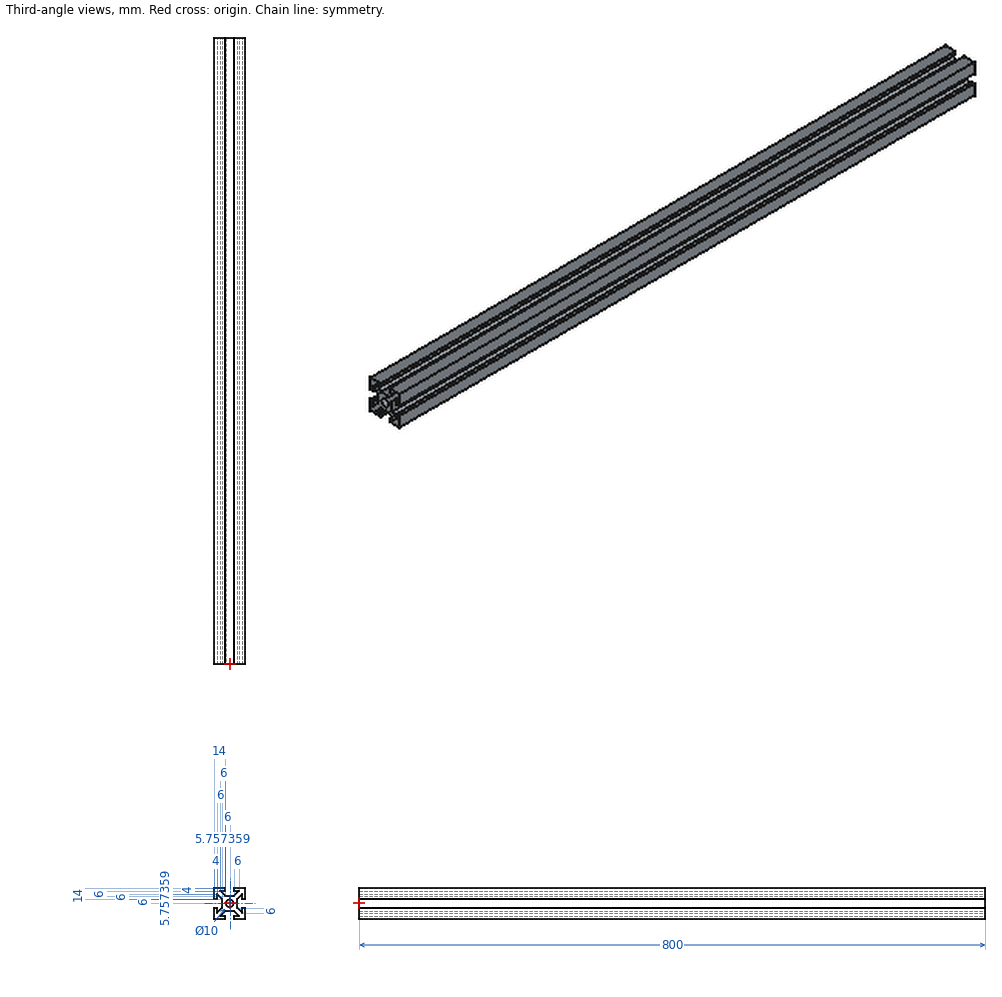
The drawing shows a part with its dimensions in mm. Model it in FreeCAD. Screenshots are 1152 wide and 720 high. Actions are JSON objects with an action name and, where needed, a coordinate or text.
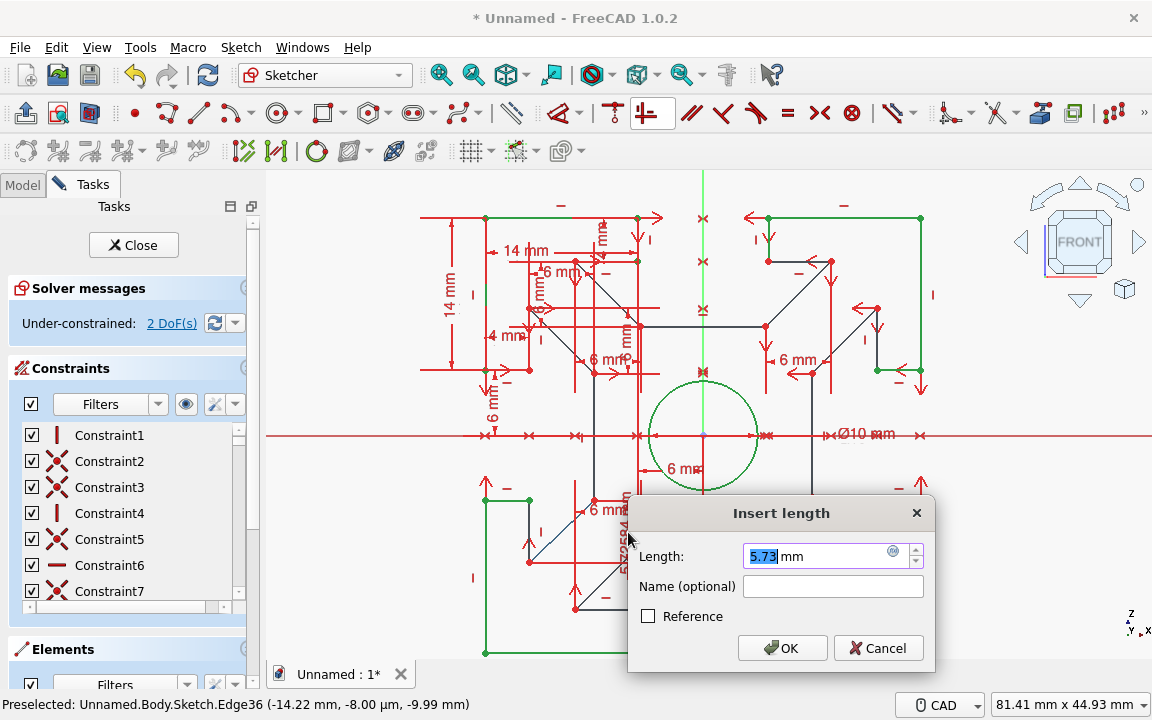
{"action": "type", "text": "6"}
{"action": "key", "text": "Return"}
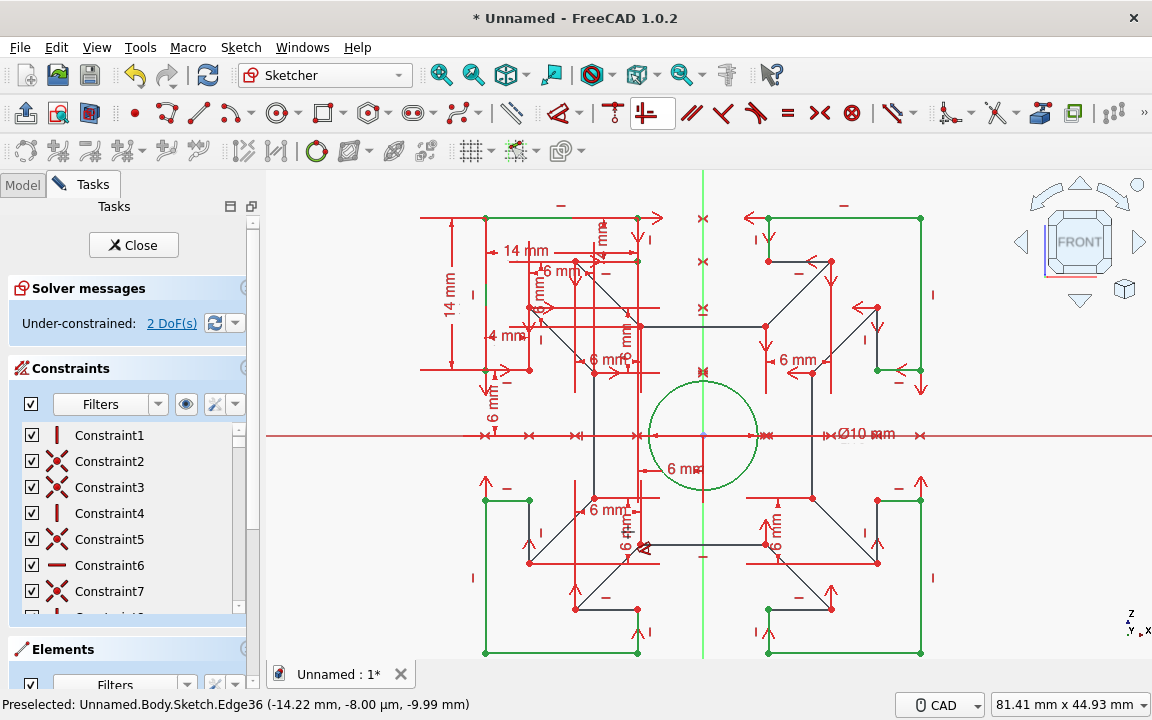
{"action": "left_click", "coordinate": [529, 327]}
{"action": "left_click", "coordinate": [471, 361]}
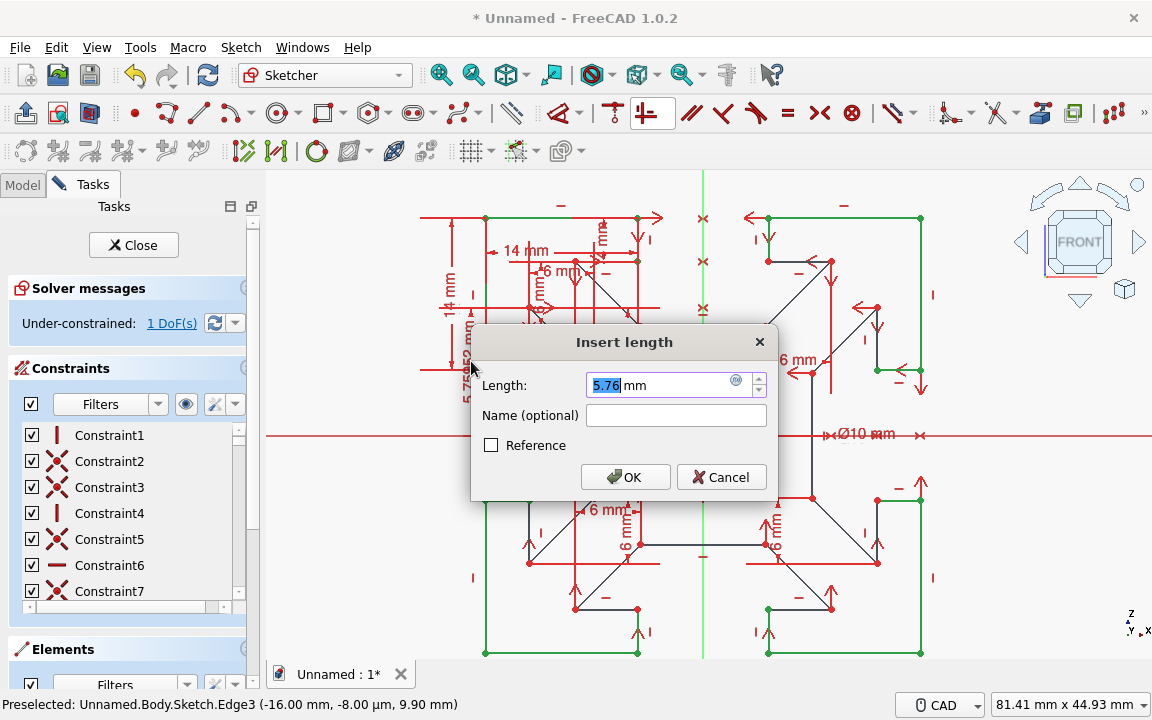
{"action": "type", "text": "5.757359"}
{"action": "key", "text": "Return"}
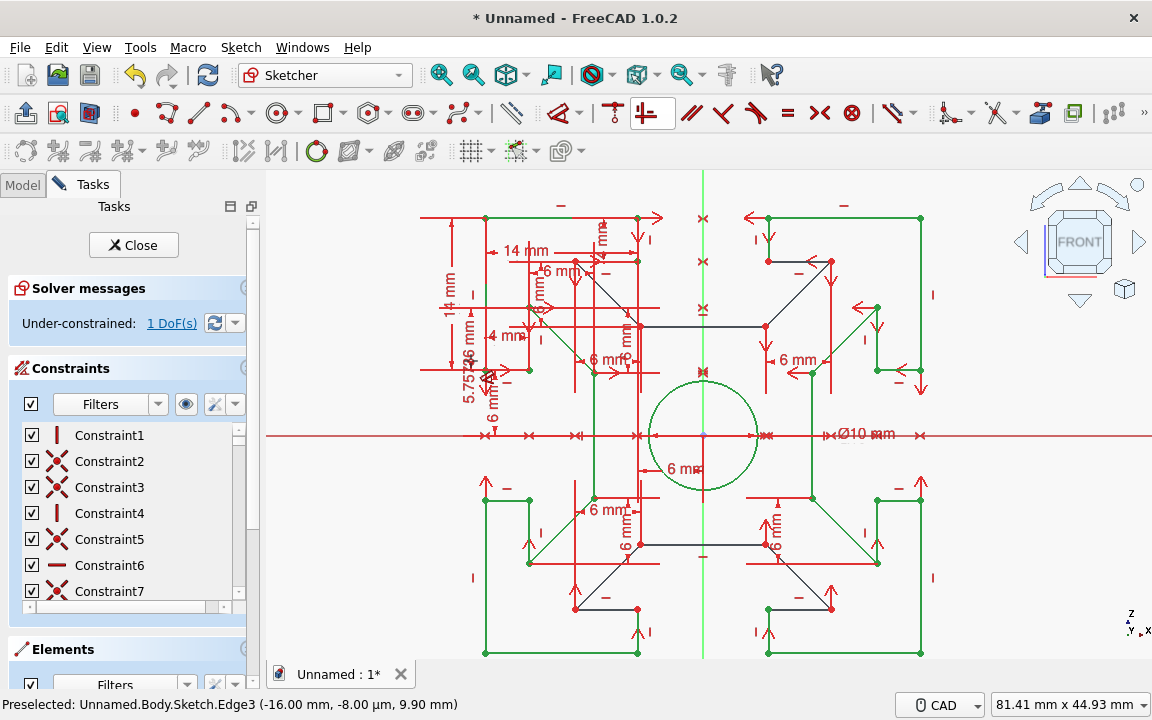
{"action": "left_click", "coordinate": [619, 262]}
{"action": "left_click", "coordinate": [629, 296]}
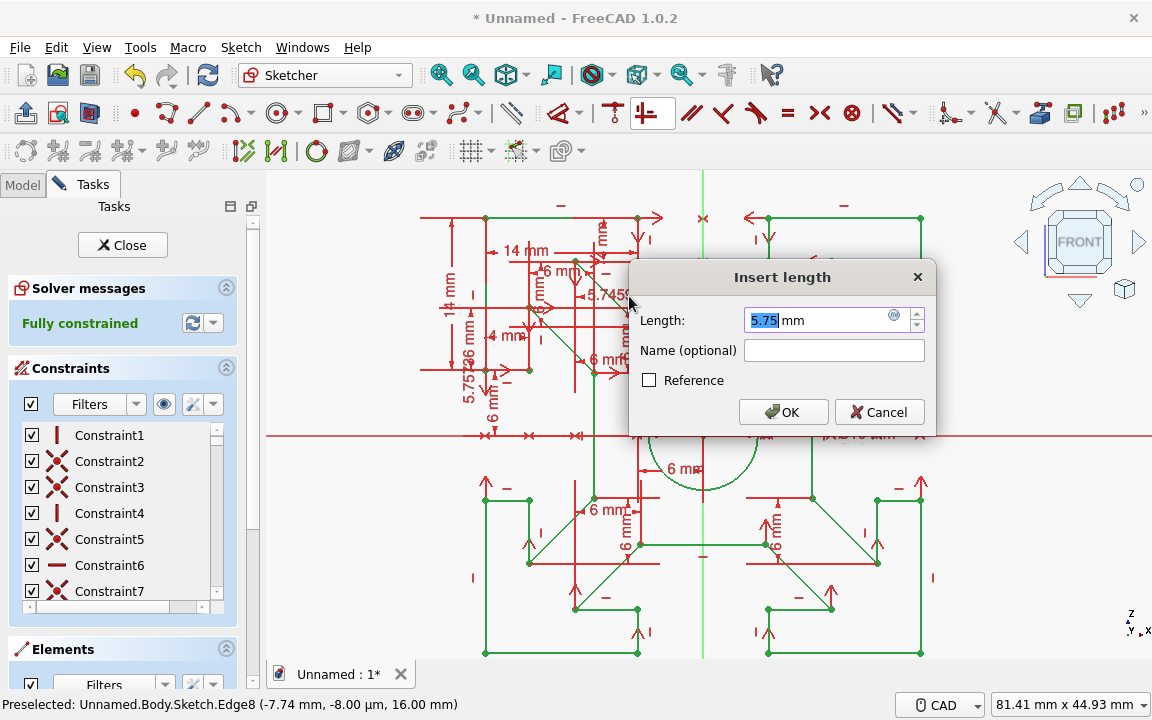
{"action": "type", "text": "5.757359"}
{"action": "key", "text": "Return"}
{"action": "key", "text": "Escape"}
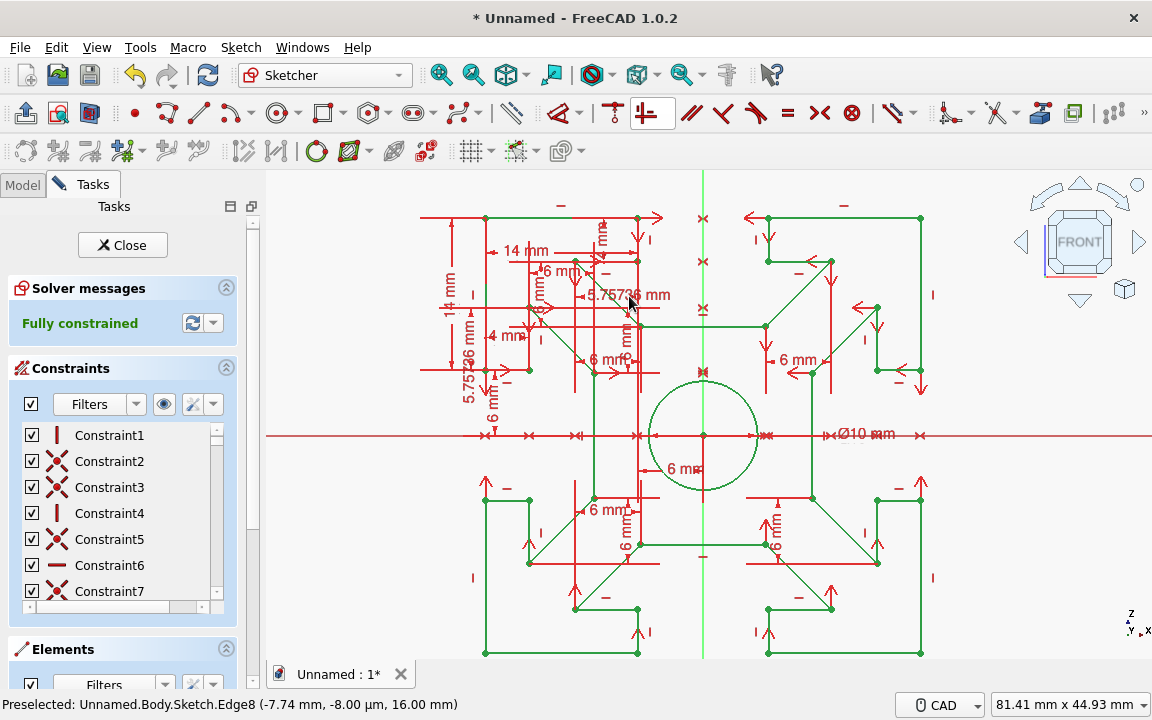
{"action": "left_click", "coordinate": [123, 245]}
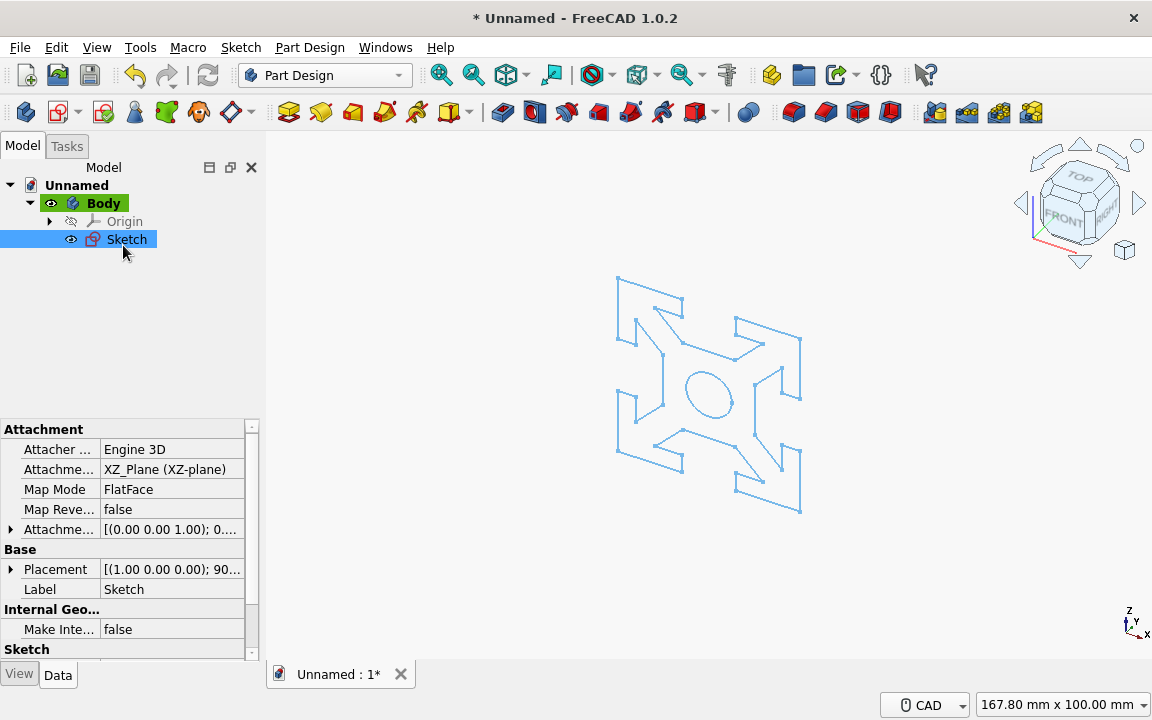
{"action": "left_click", "coordinate": [290, 112]}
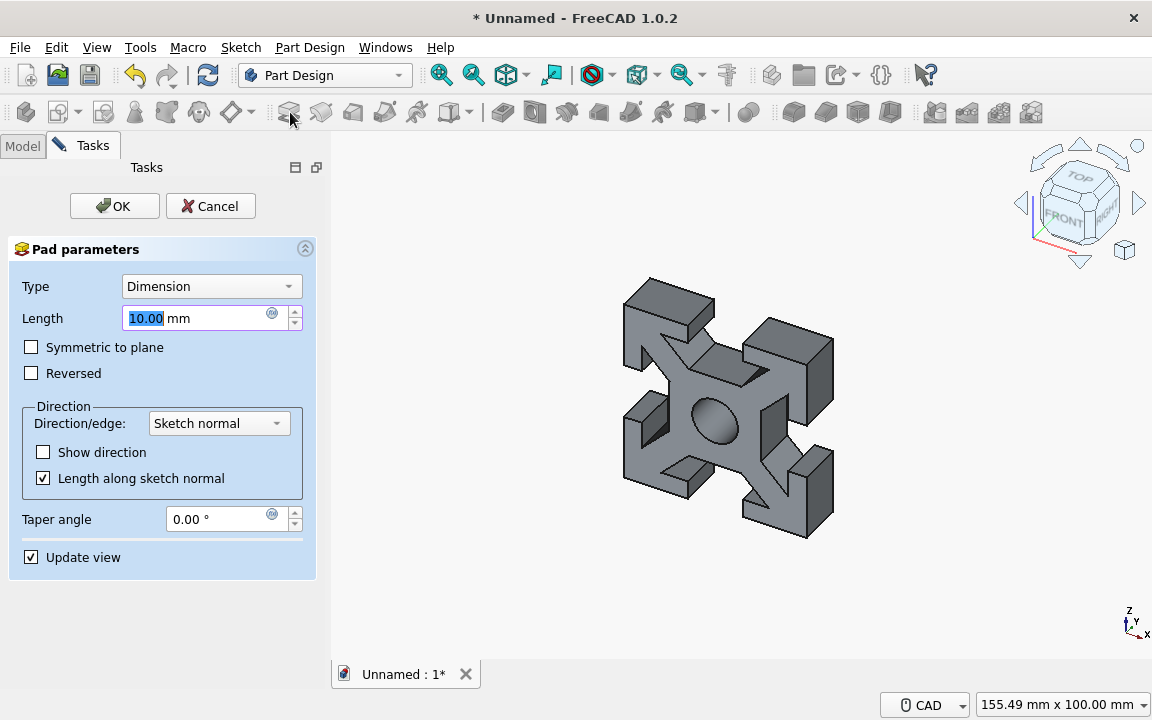
{"action": "type", "text": "800"}
{"action": "key", "text": "Tab"}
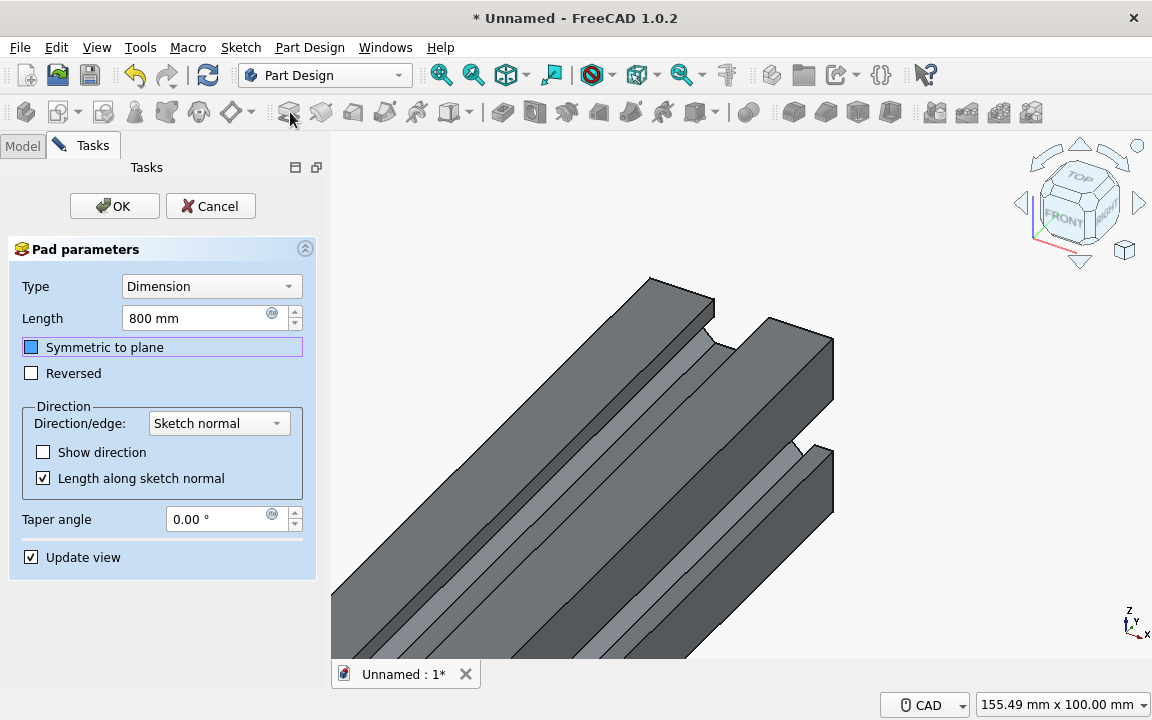
{"action": "left_click", "coordinate": [30, 373]}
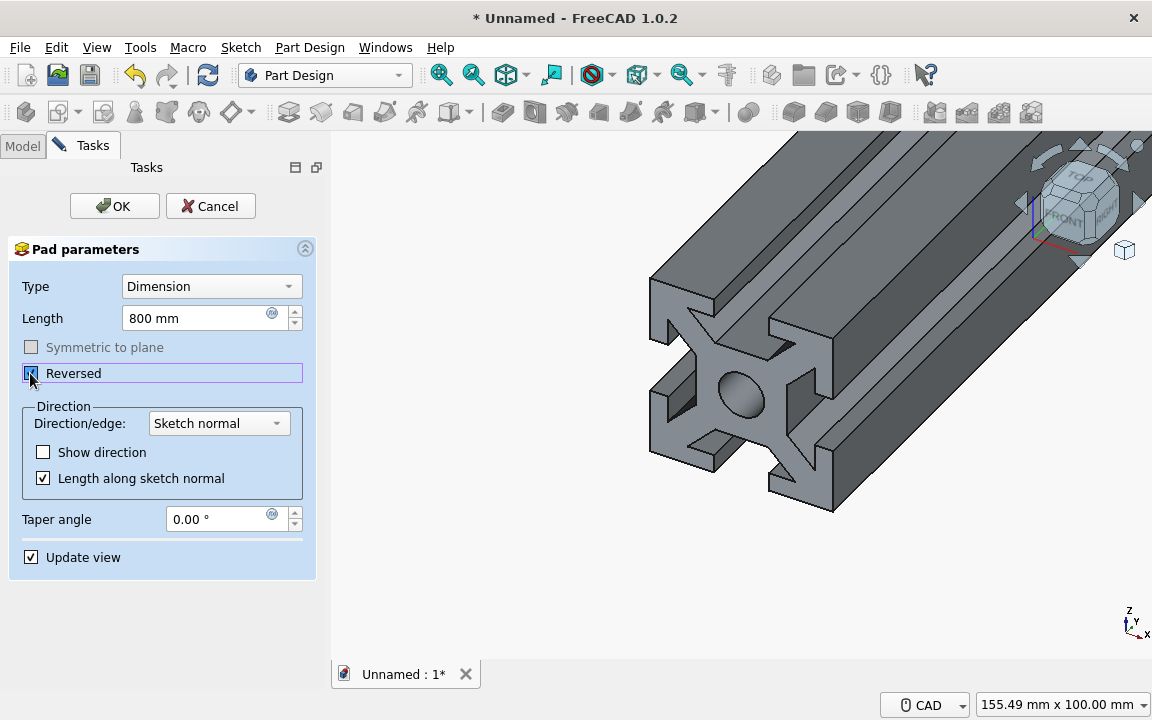
{"action": "left_click", "coordinate": [115, 206]}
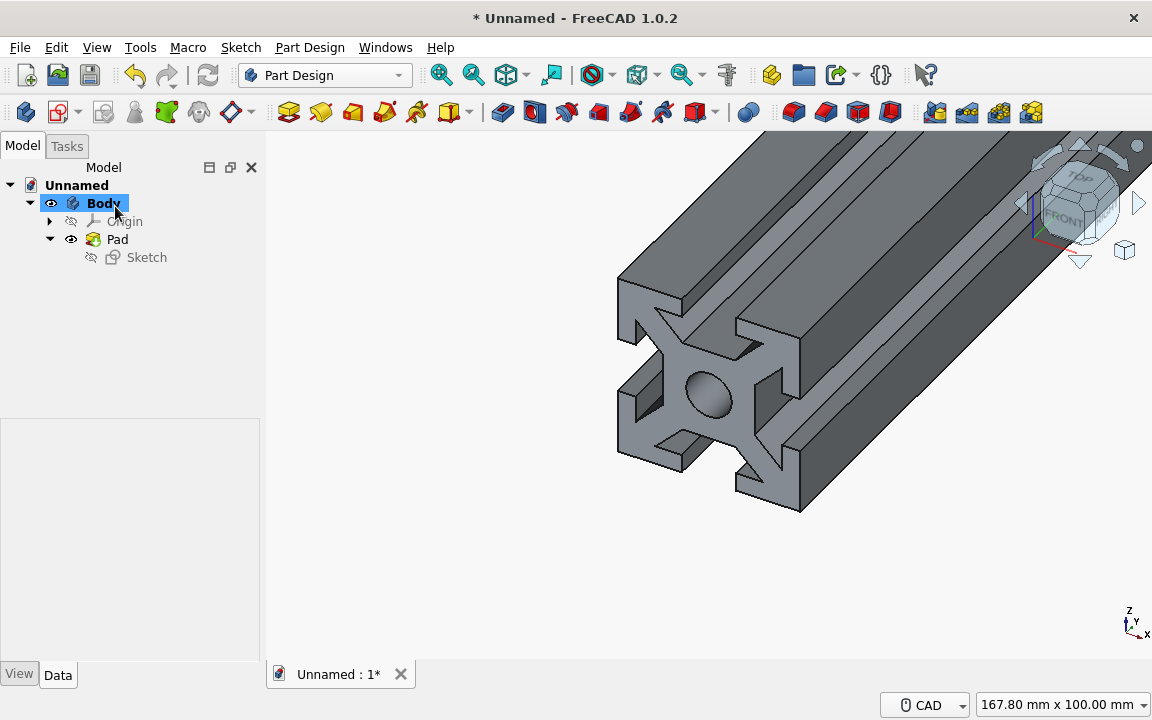
{"action": "key", "text": "0"}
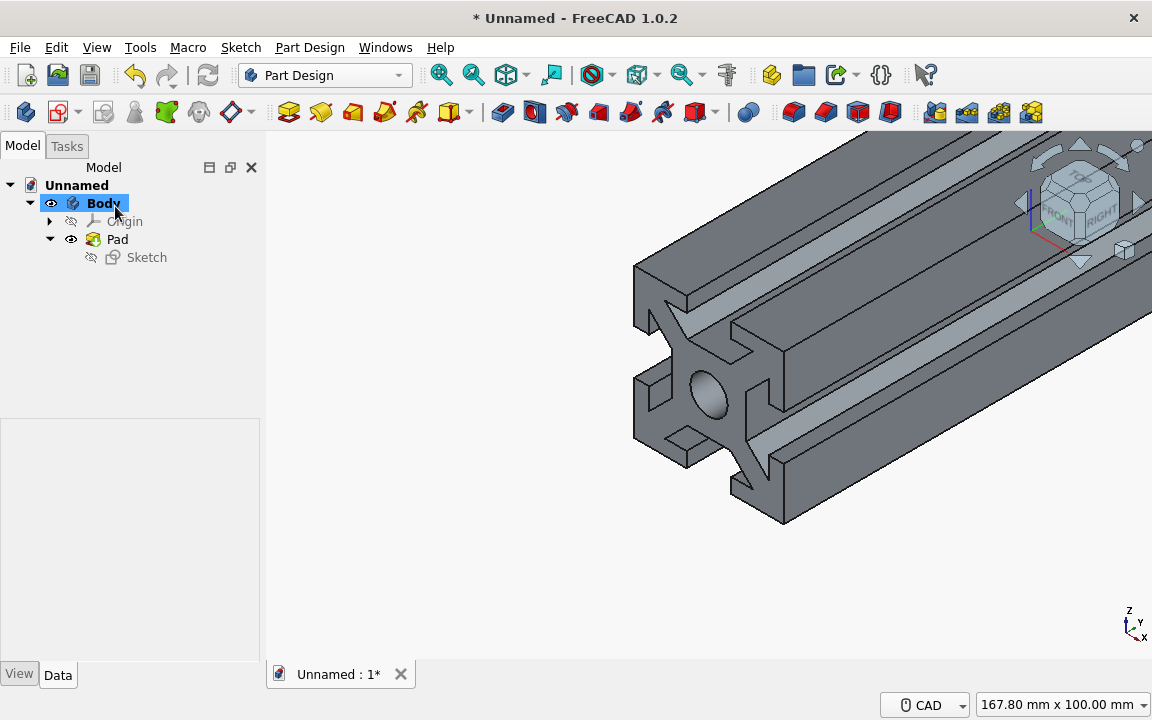
{"action": "left_click", "coordinate": [442, 76]}